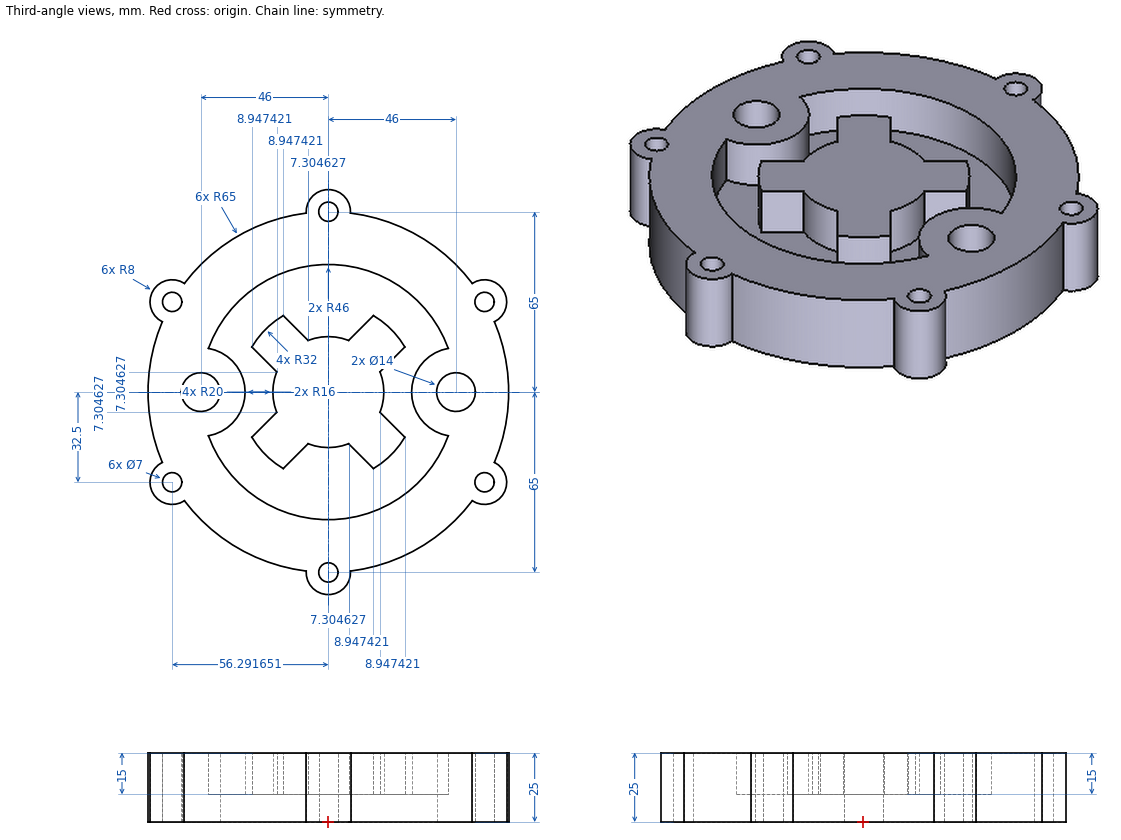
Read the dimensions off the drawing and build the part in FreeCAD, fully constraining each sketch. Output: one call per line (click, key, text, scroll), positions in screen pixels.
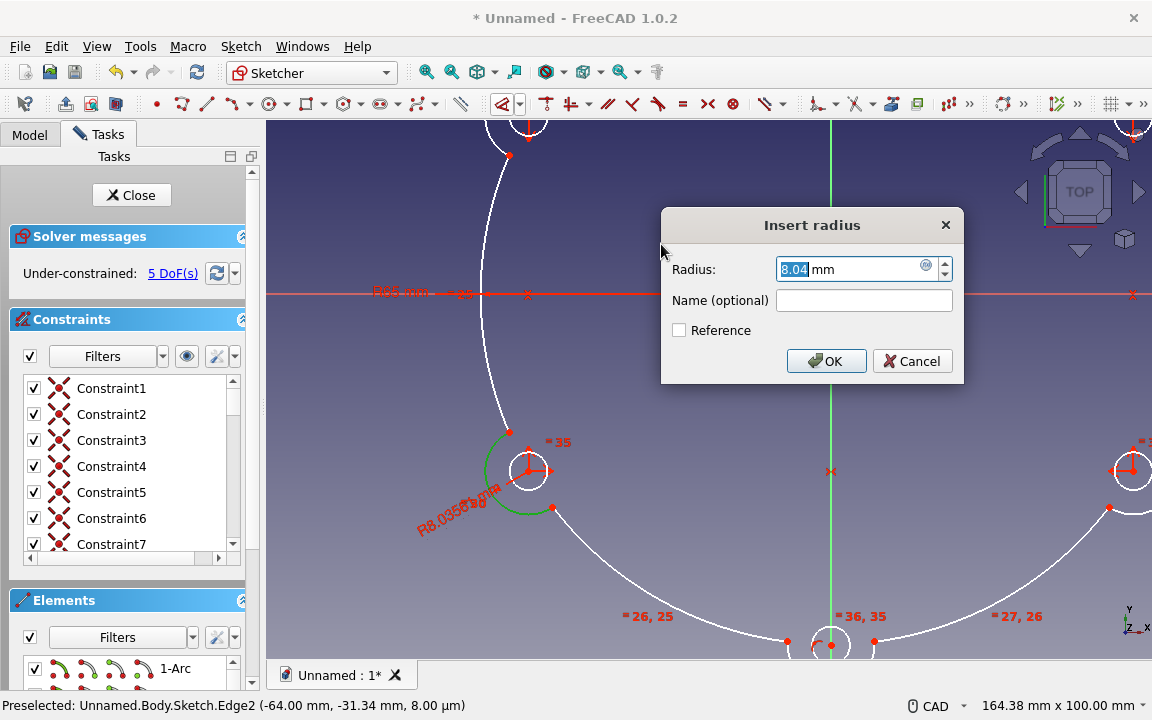
text(8)
key(Return)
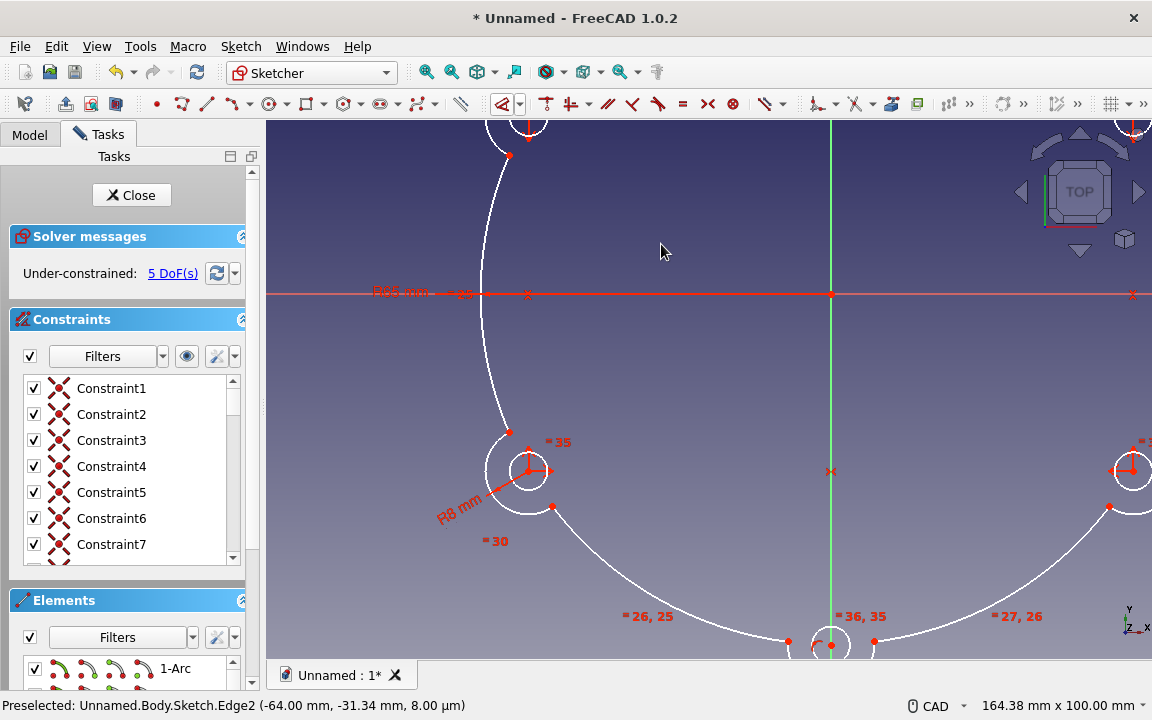
click(542, 458)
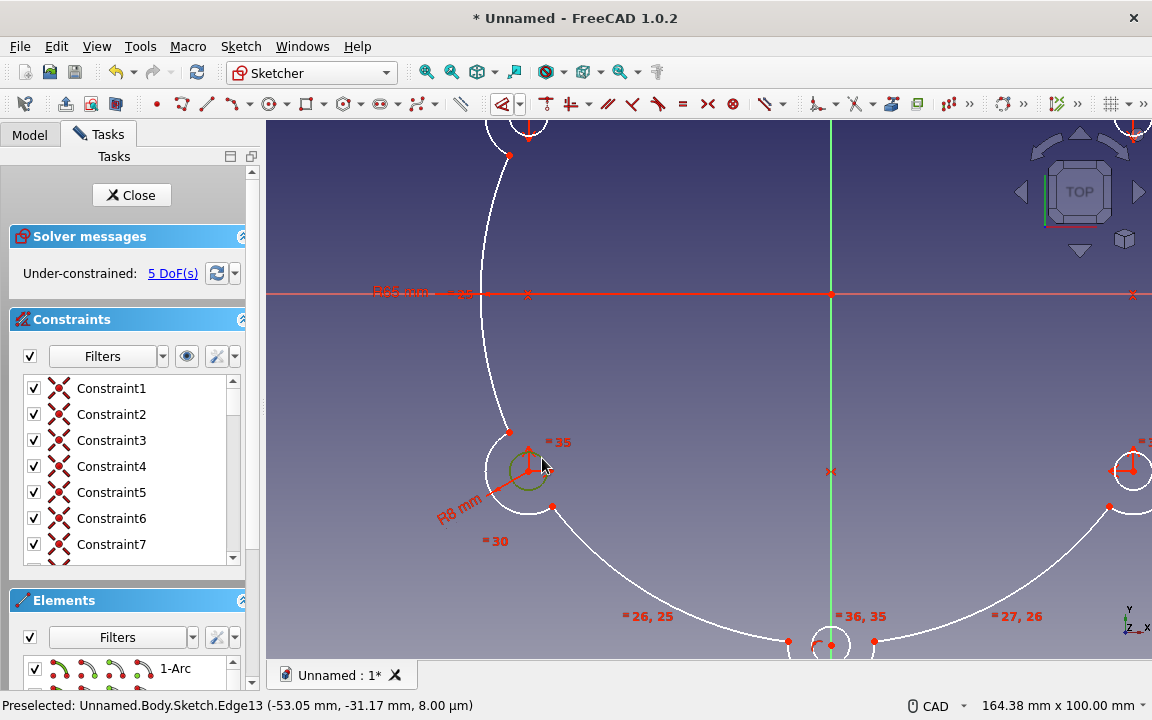
key(k)
key(o)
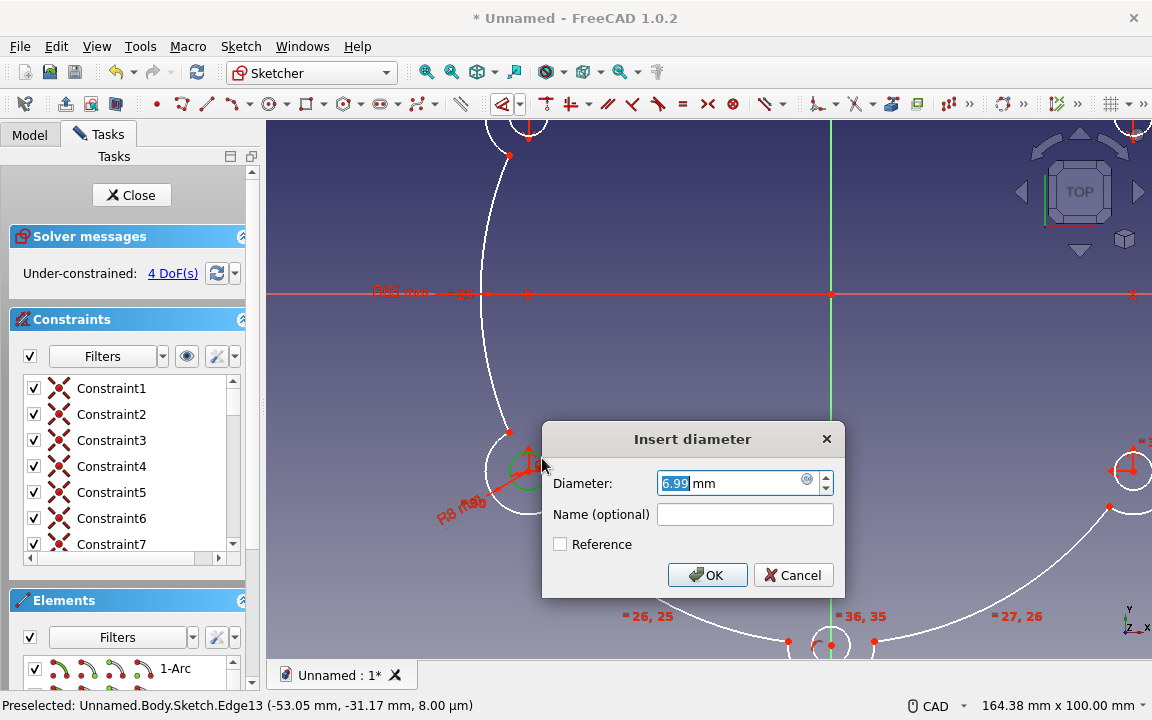
text(7)
key(Return)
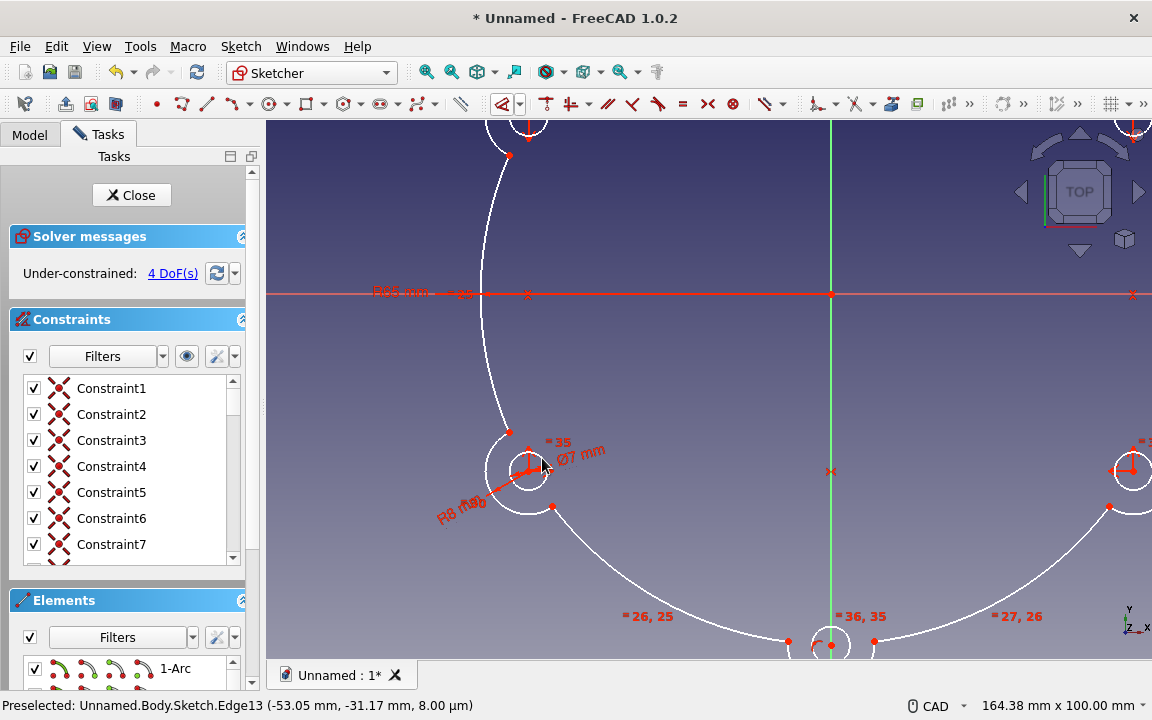
scroll(485, 467, down, 4)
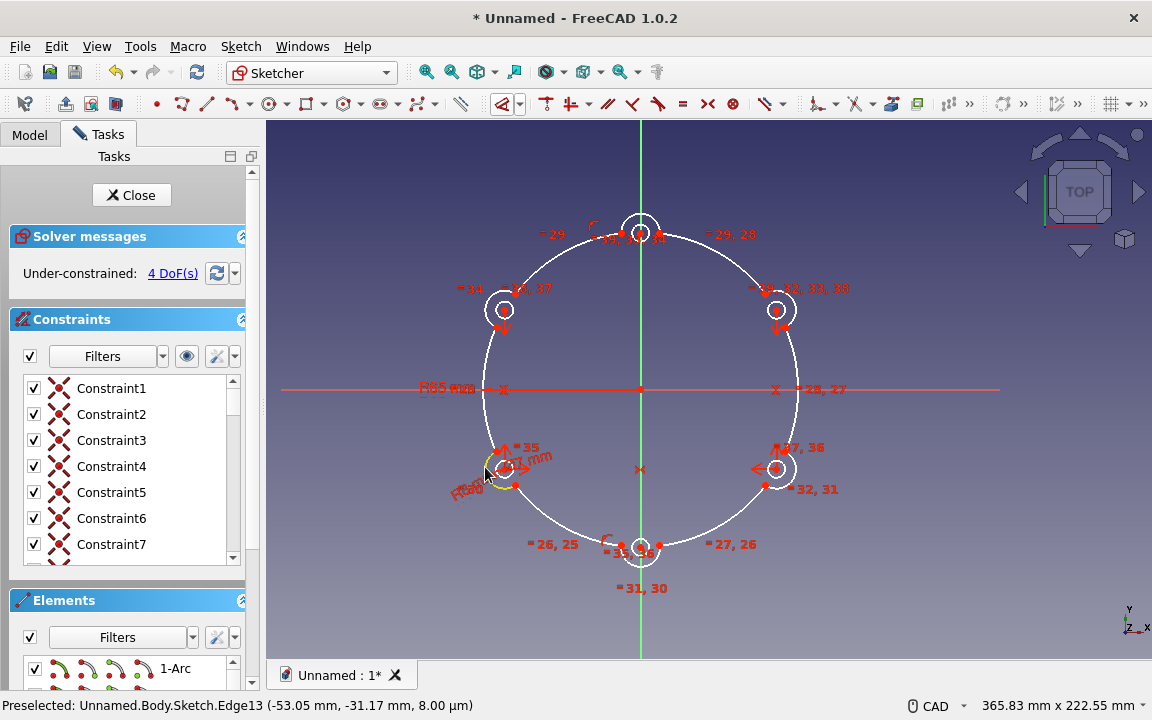
click(641, 547)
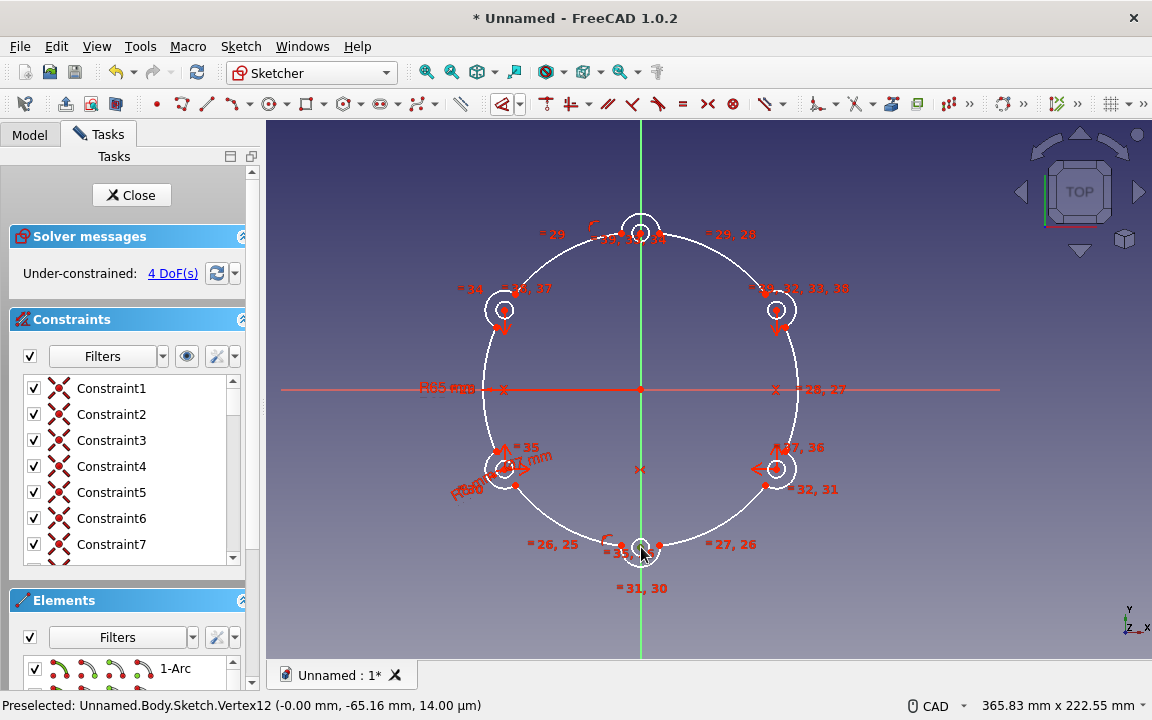
key(i)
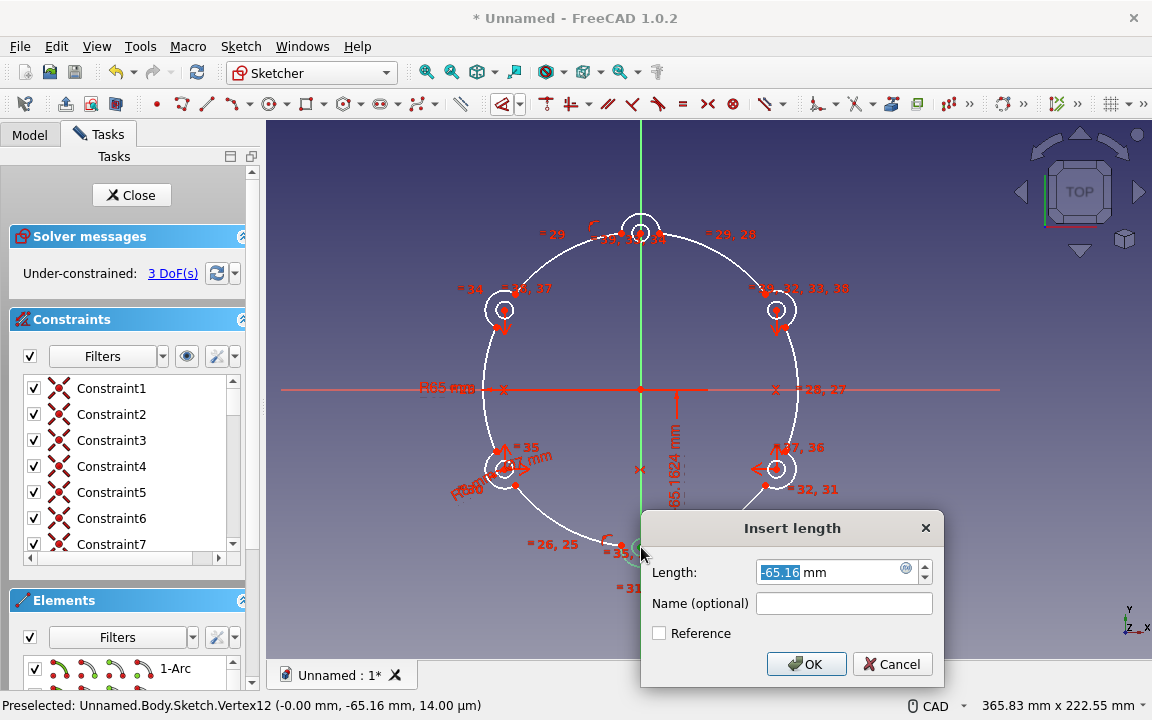
text(-65)
key(Return)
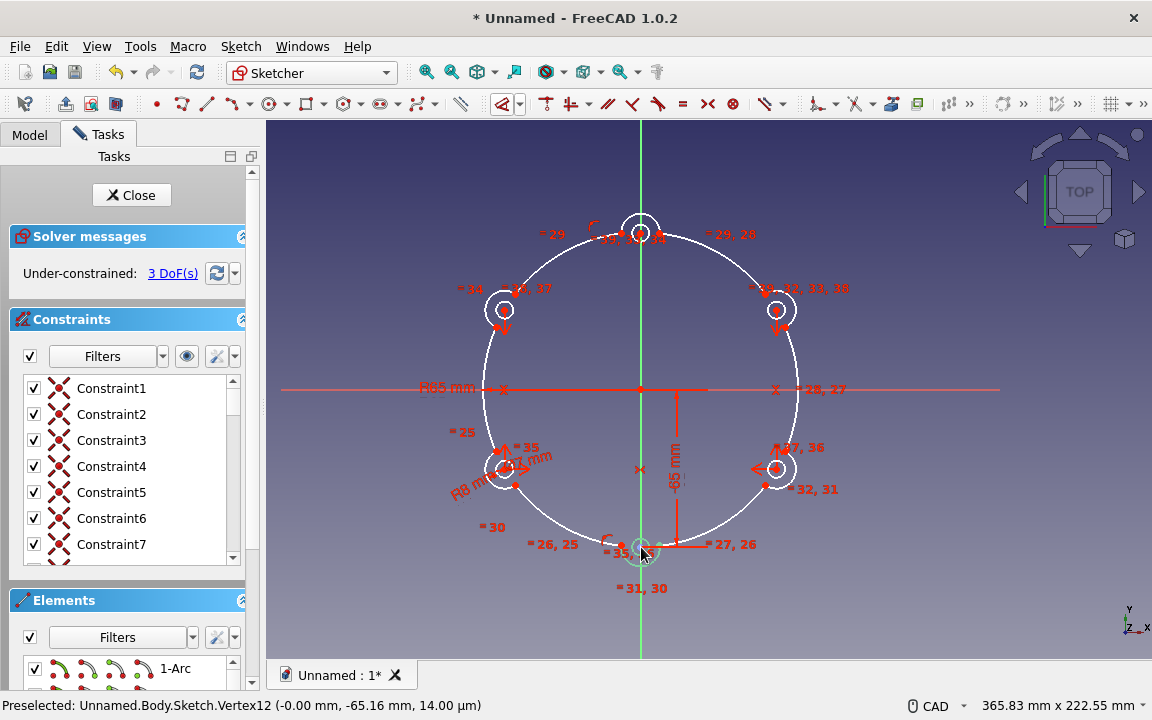
click(641, 233)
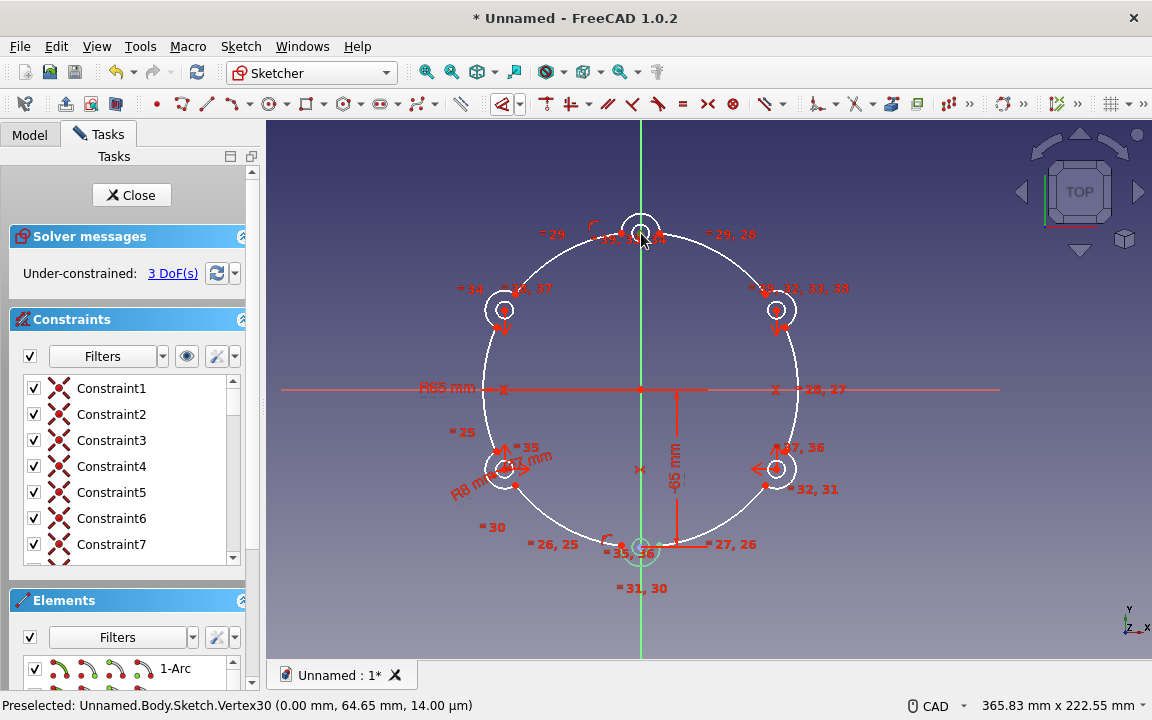
key(i)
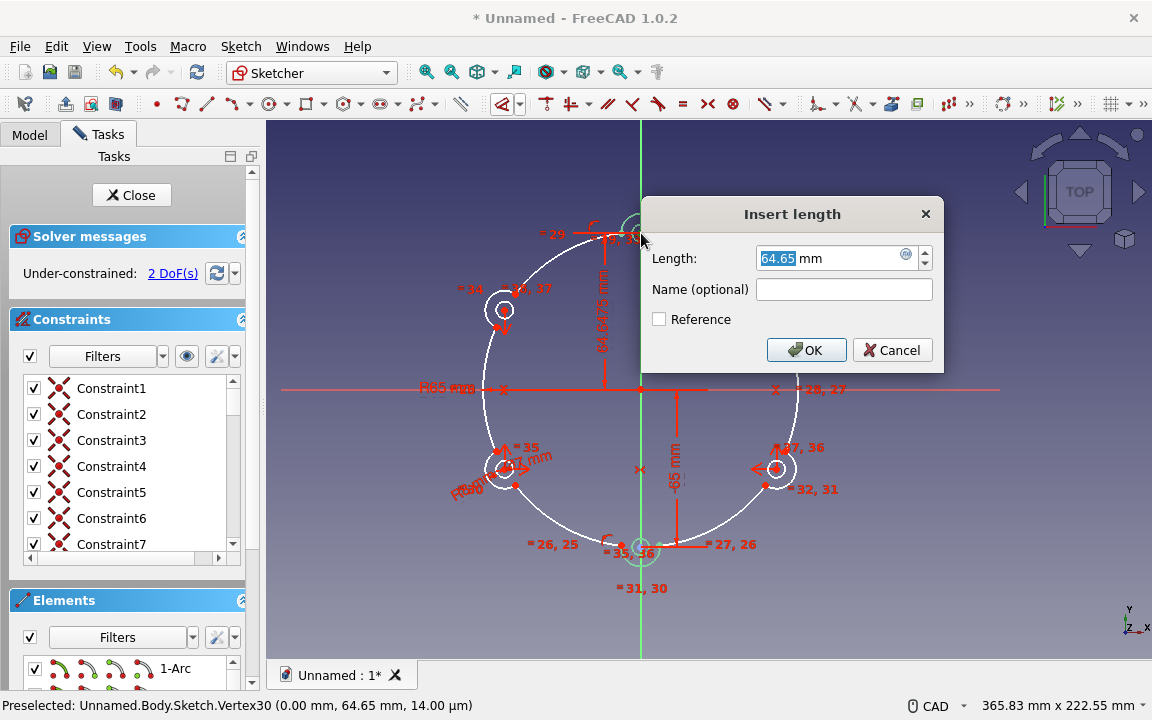
text(65)
key(Return)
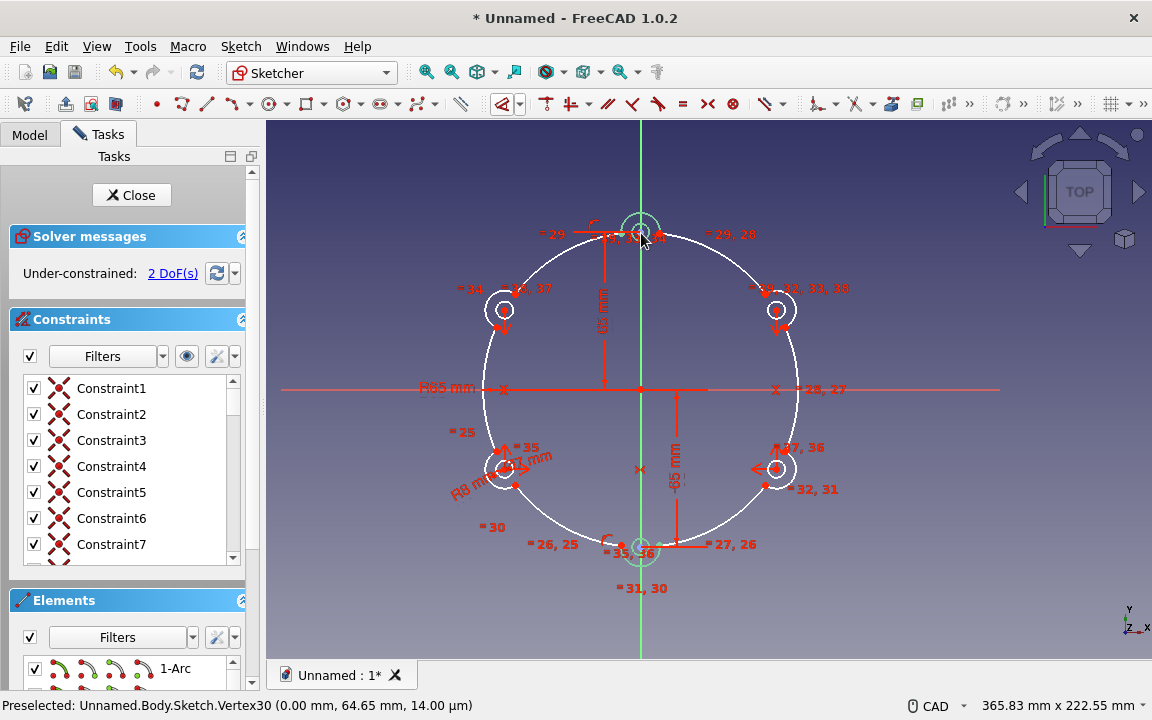
click(505, 469)